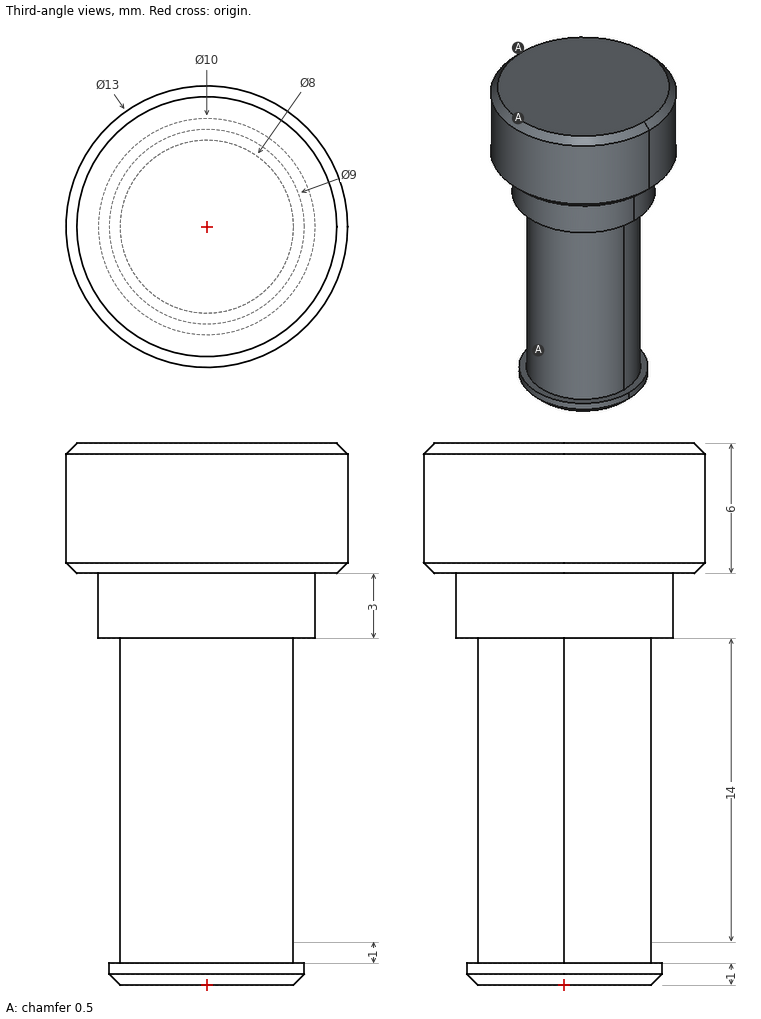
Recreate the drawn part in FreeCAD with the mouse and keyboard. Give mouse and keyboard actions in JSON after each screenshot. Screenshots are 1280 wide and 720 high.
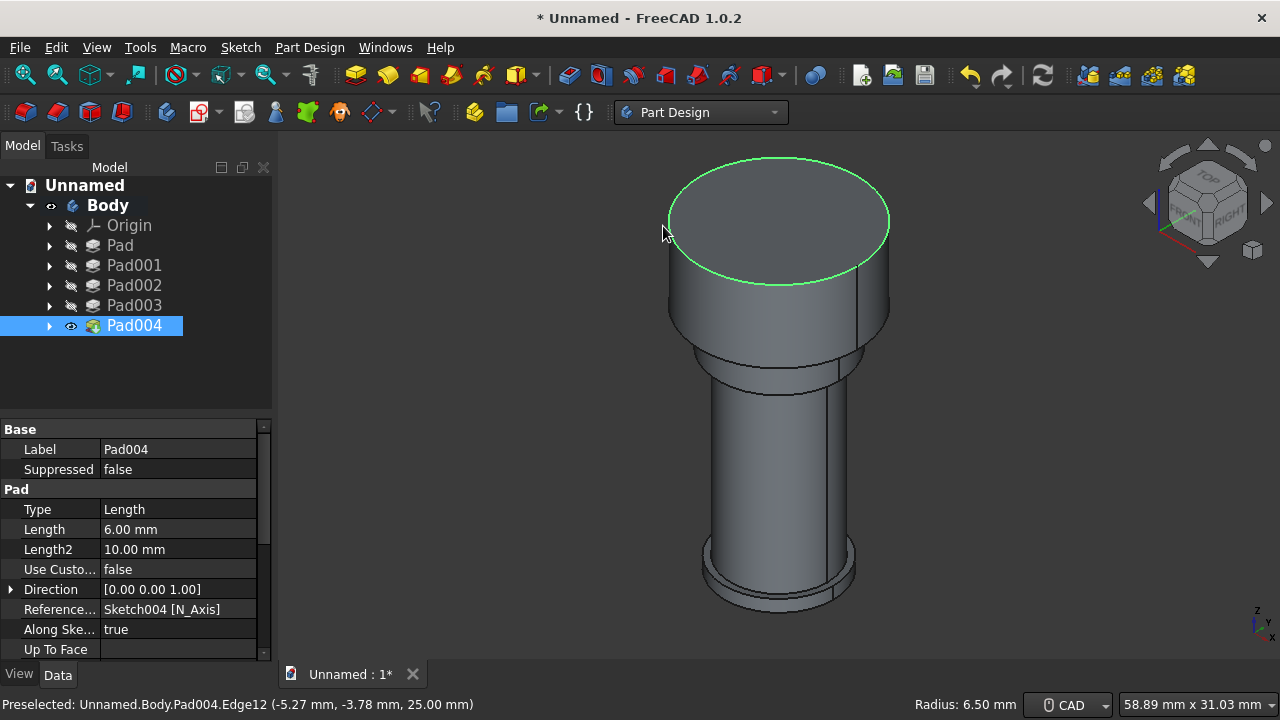
{"action": "left_click", "coordinate": [26, 76]}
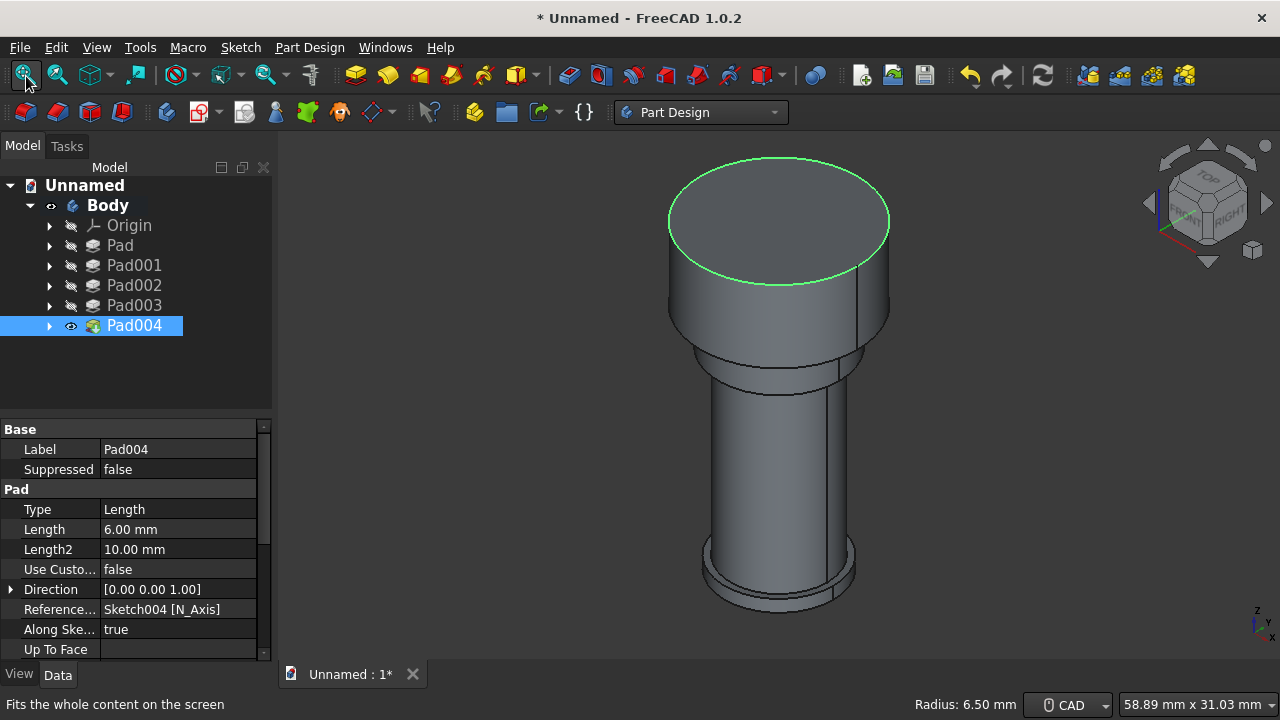
{"action": "left_click", "coordinate": [680, 333], "text": "ctrl"}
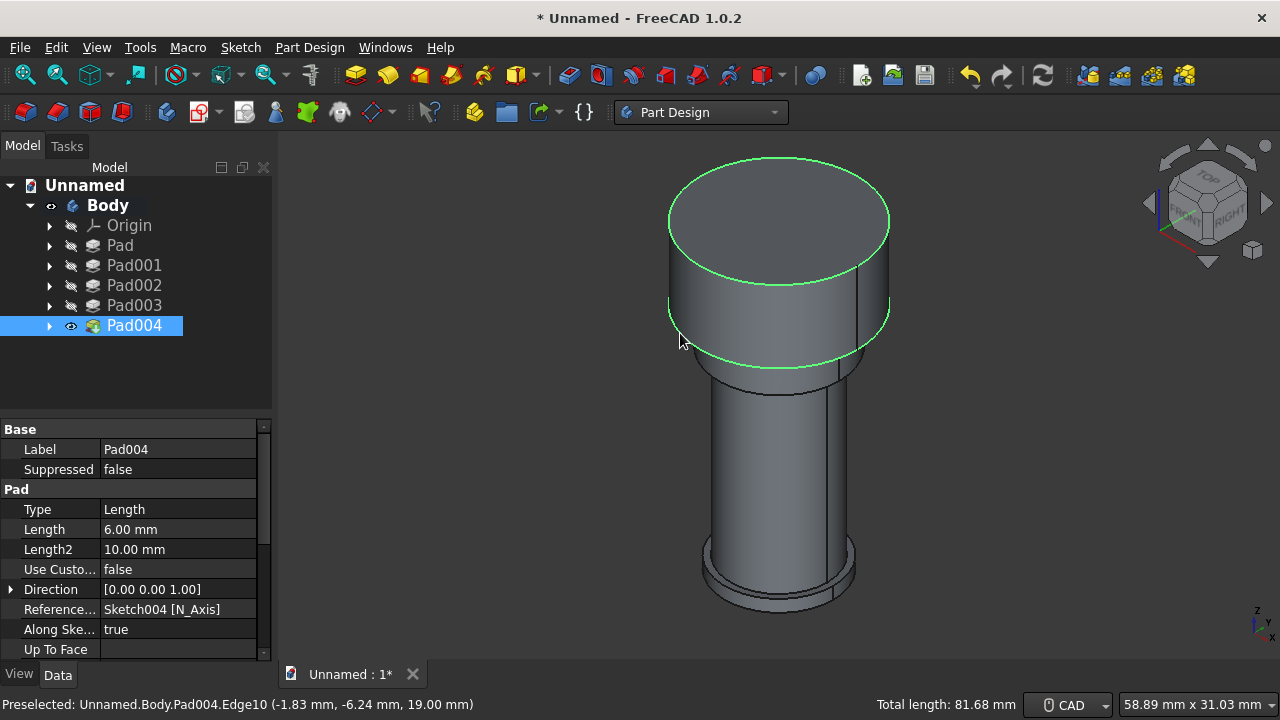
{"action": "key", "text": "2"}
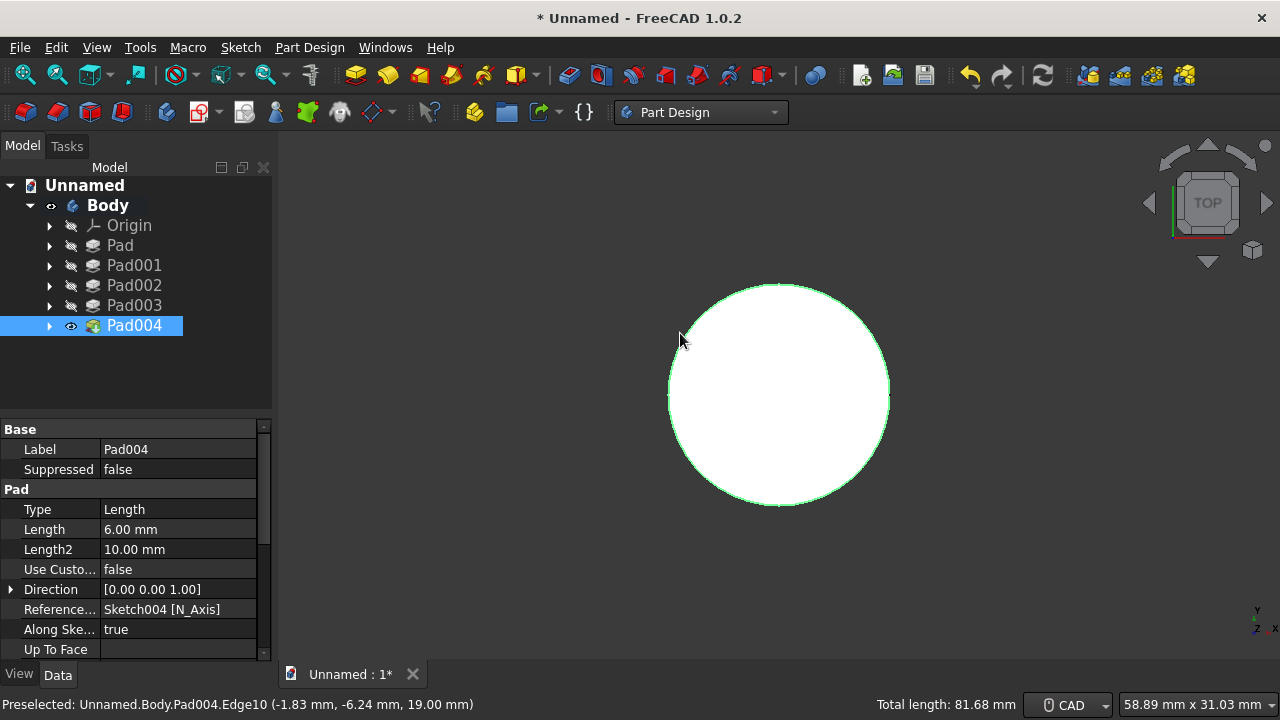
{"action": "left_click", "coordinate": [26, 76]}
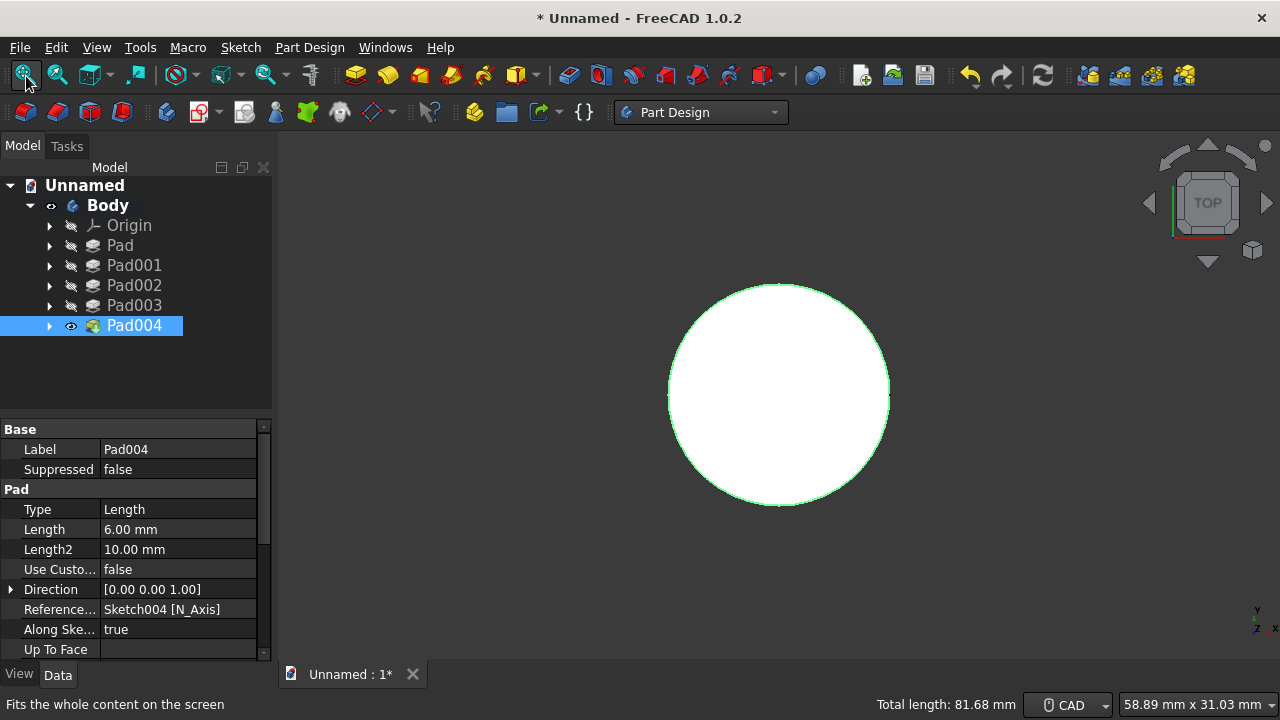
{"action": "key", "text": "1"}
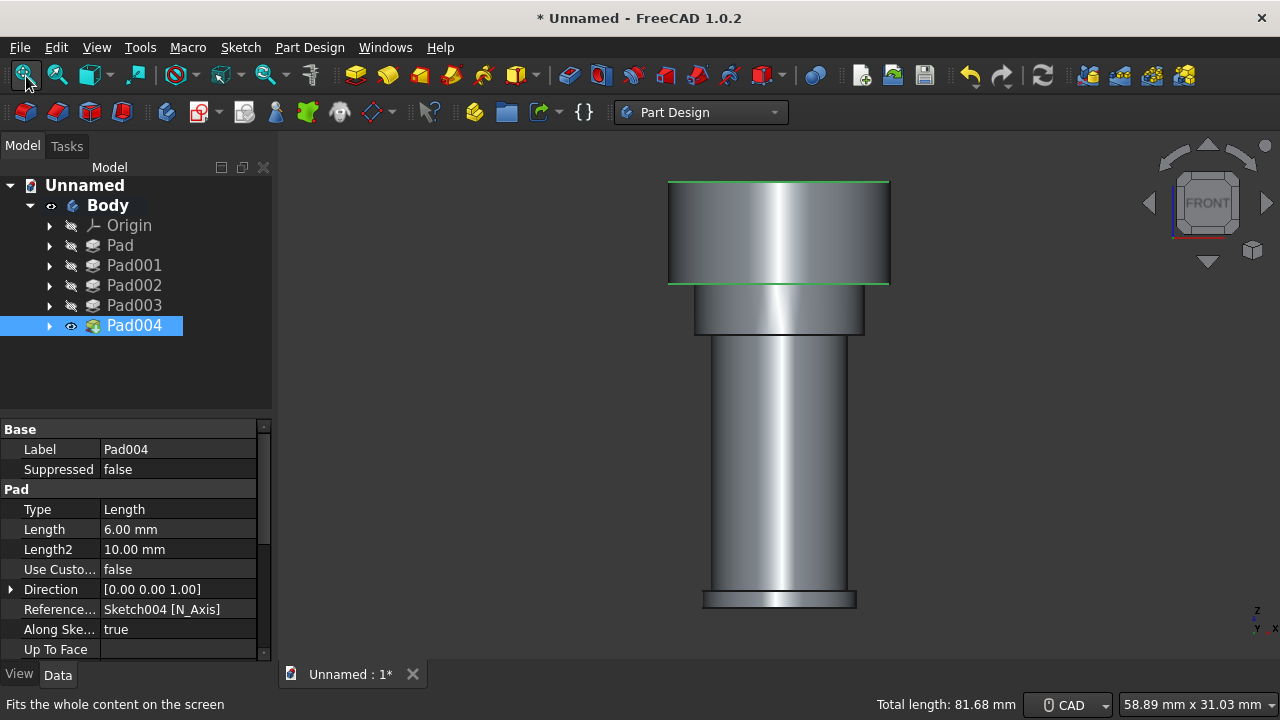
{"action": "left_click", "coordinate": [717, 607], "text": "ctrl"}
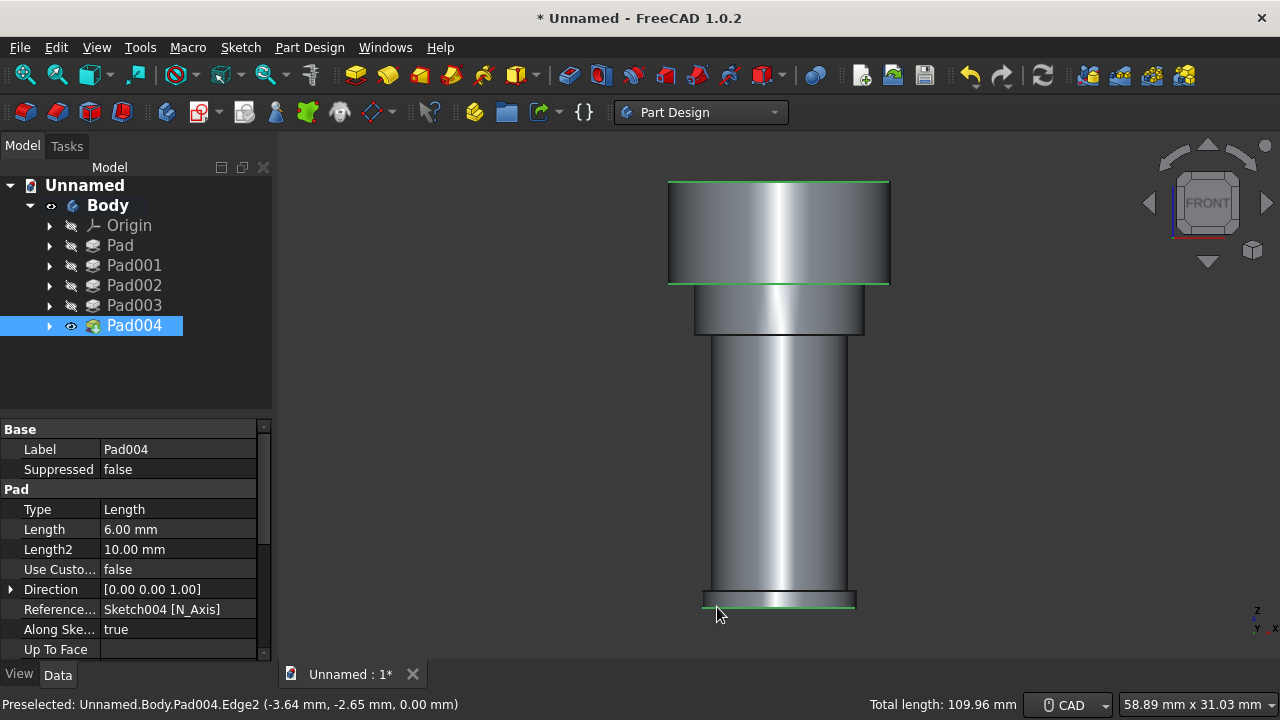
{"action": "left_click", "coordinate": [58, 112]}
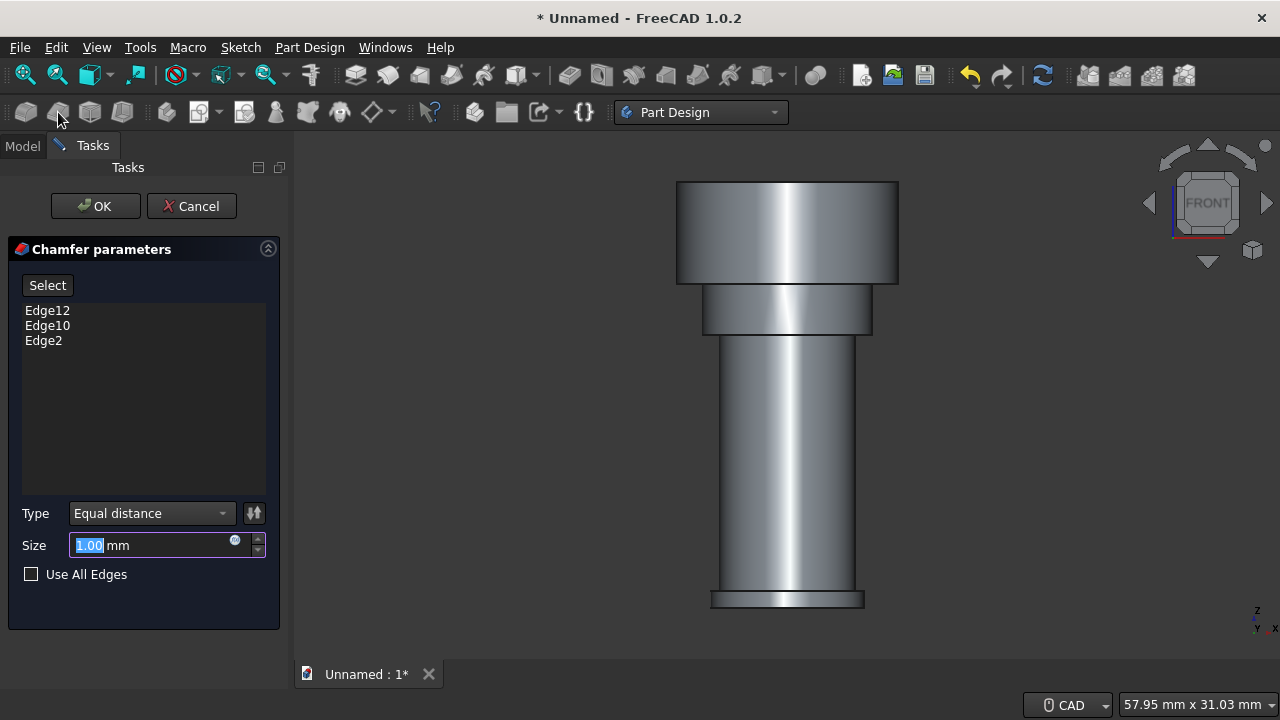
{"action": "type", "text": "0.5"}
{"action": "key", "text": "Tab"}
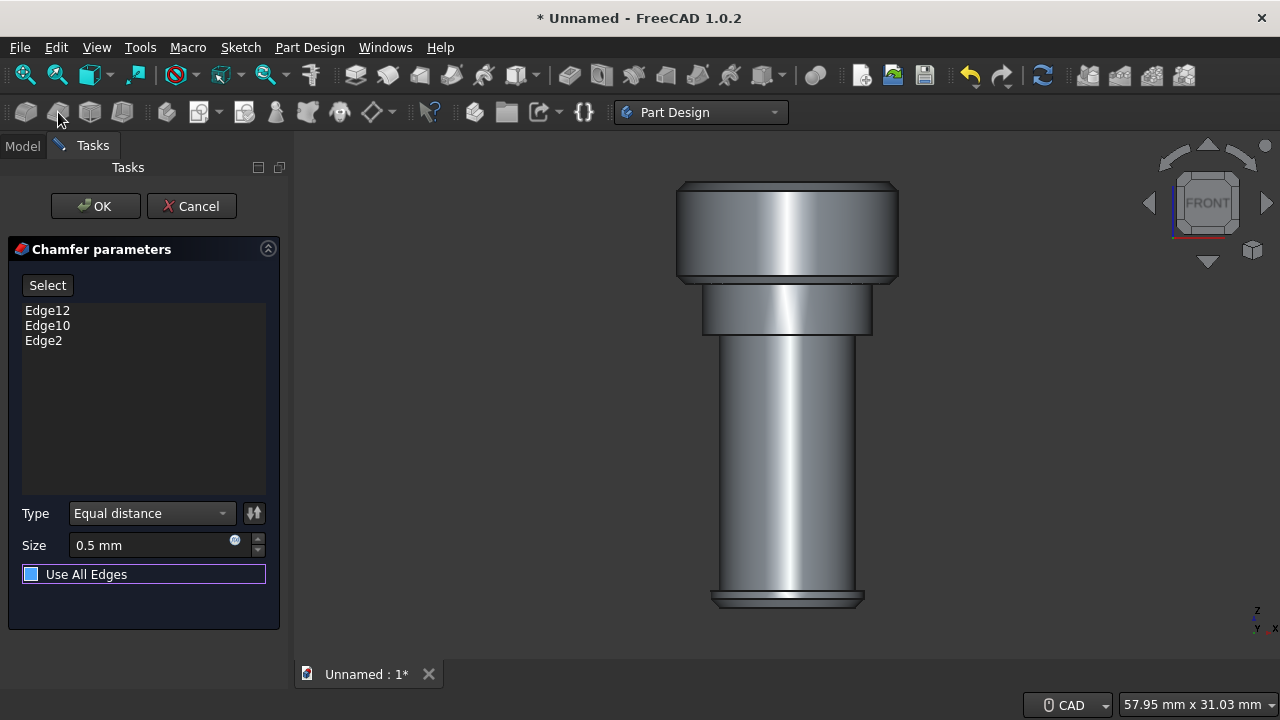
{"action": "left_click", "coordinate": [96, 206]}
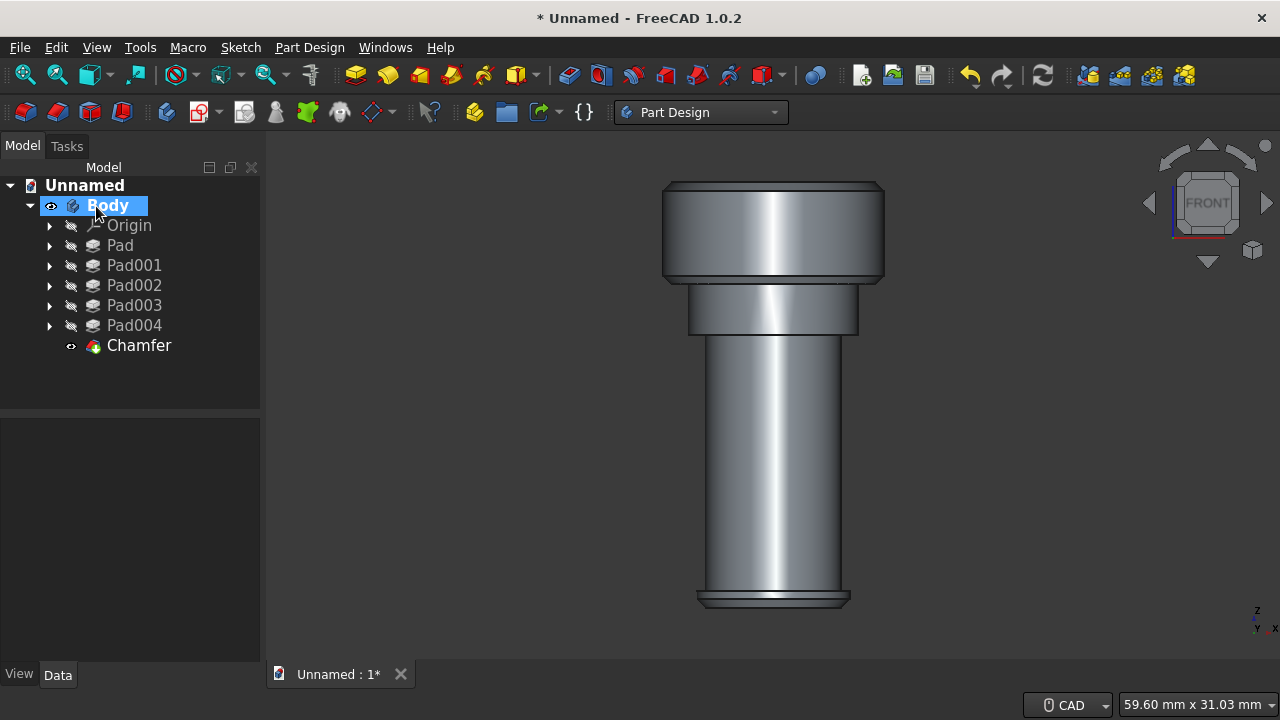
{"action": "key", "text": "0"}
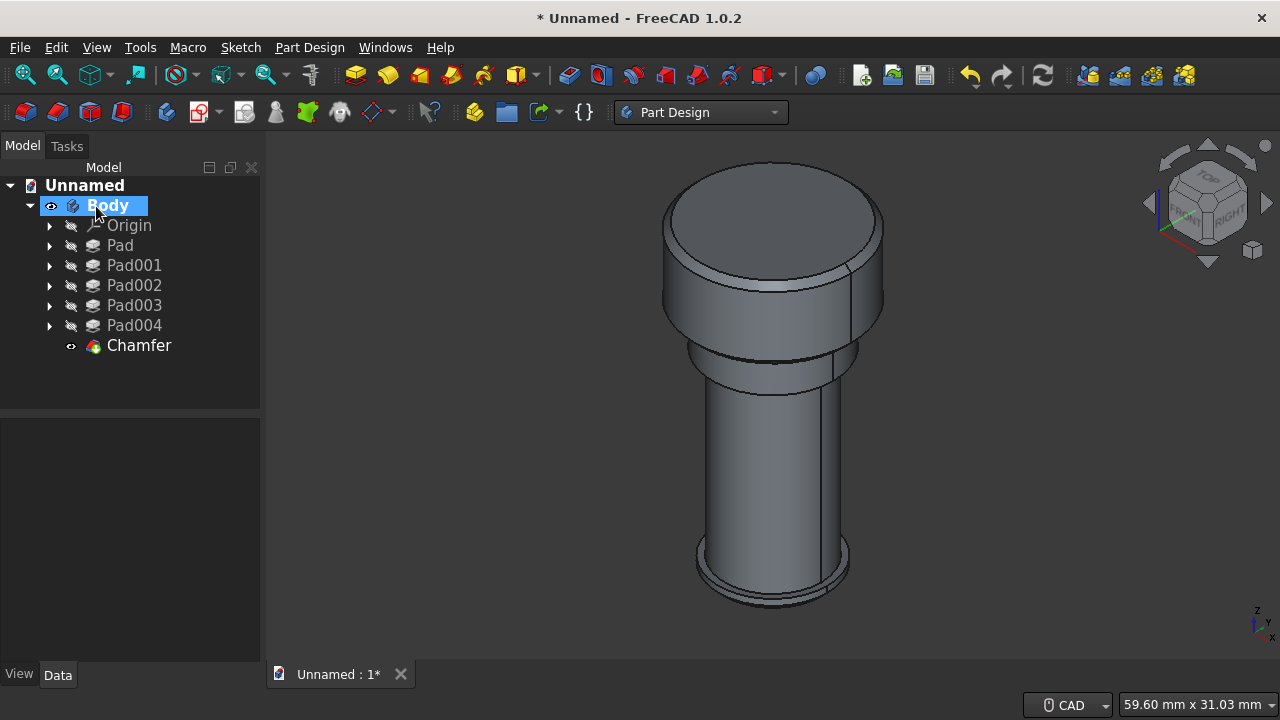
{"action": "left_click", "coordinate": [26, 76]}